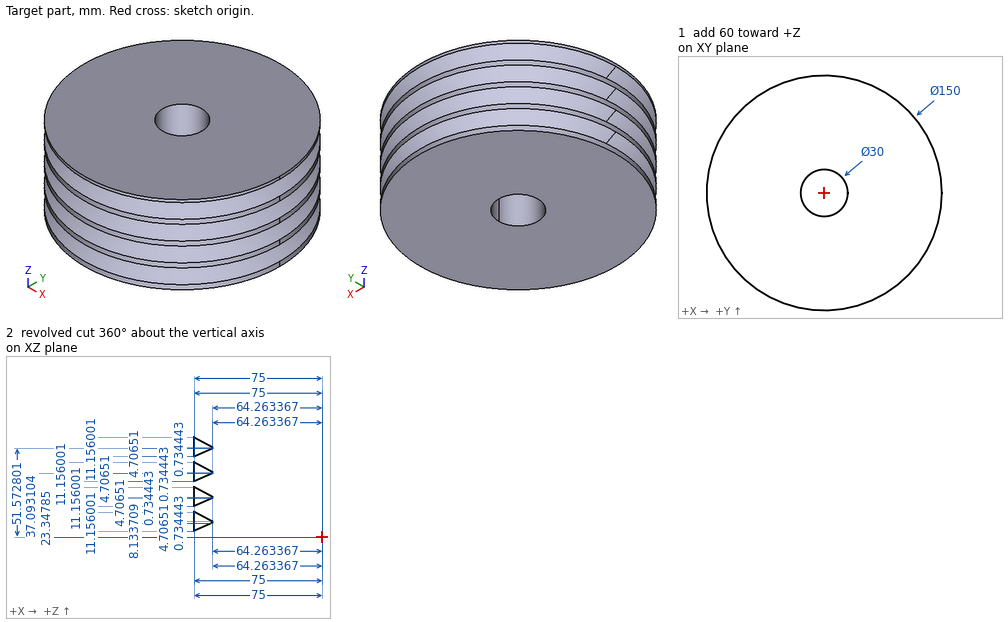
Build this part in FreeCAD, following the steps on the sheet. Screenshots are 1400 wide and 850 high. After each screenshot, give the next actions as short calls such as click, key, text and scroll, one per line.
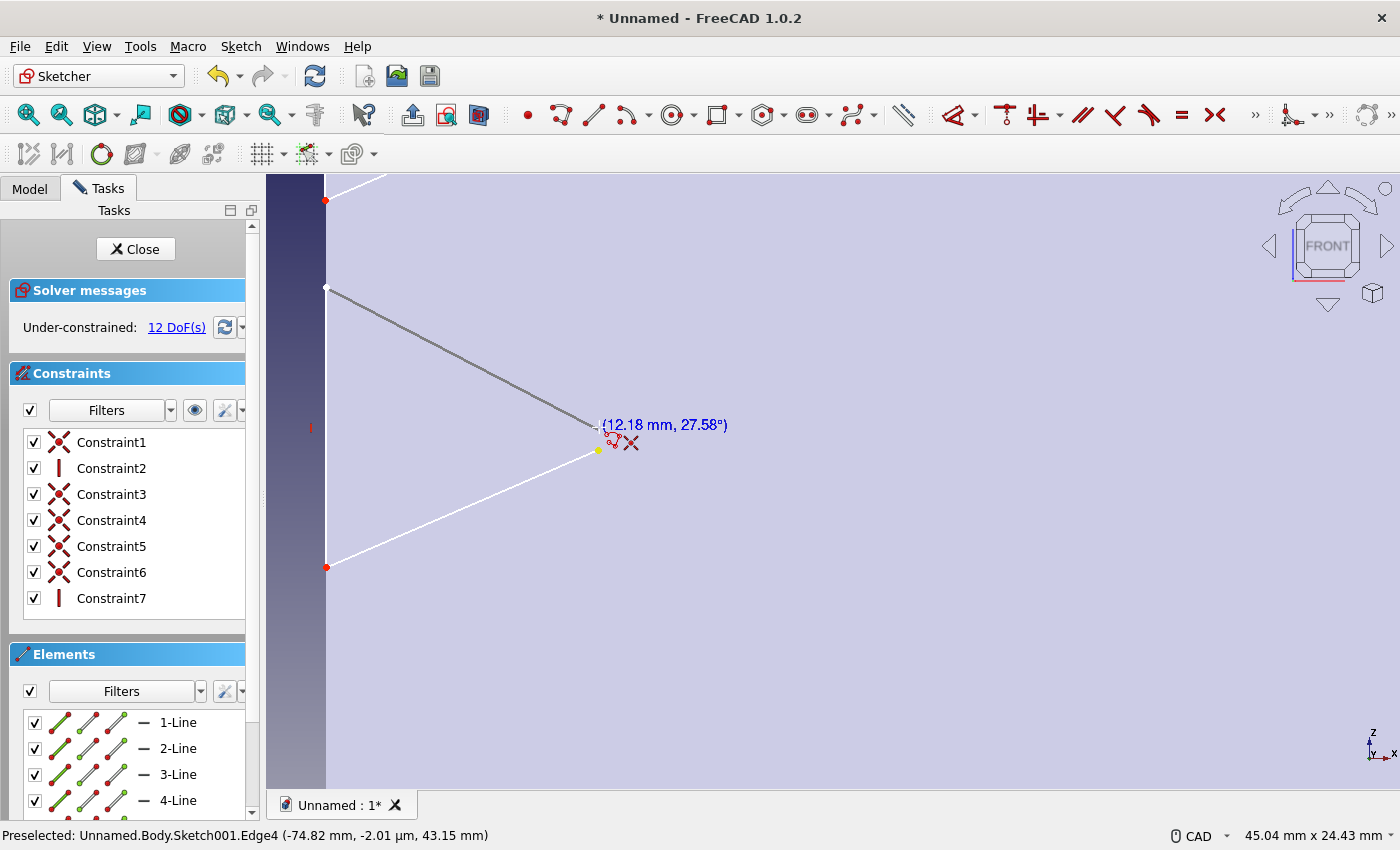
click(596, 426)
click(598, 450)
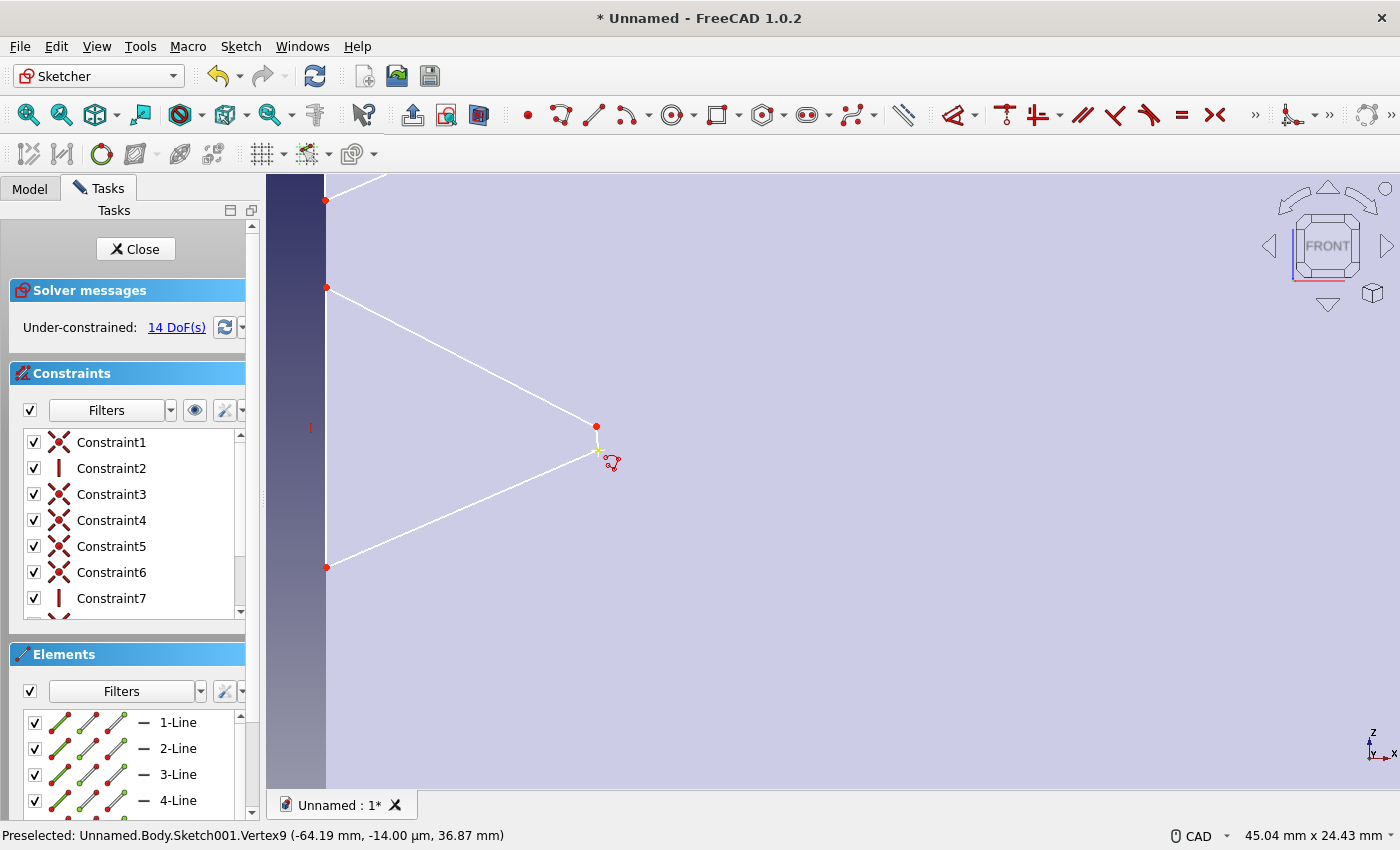
scroll(599, 427, down, 7)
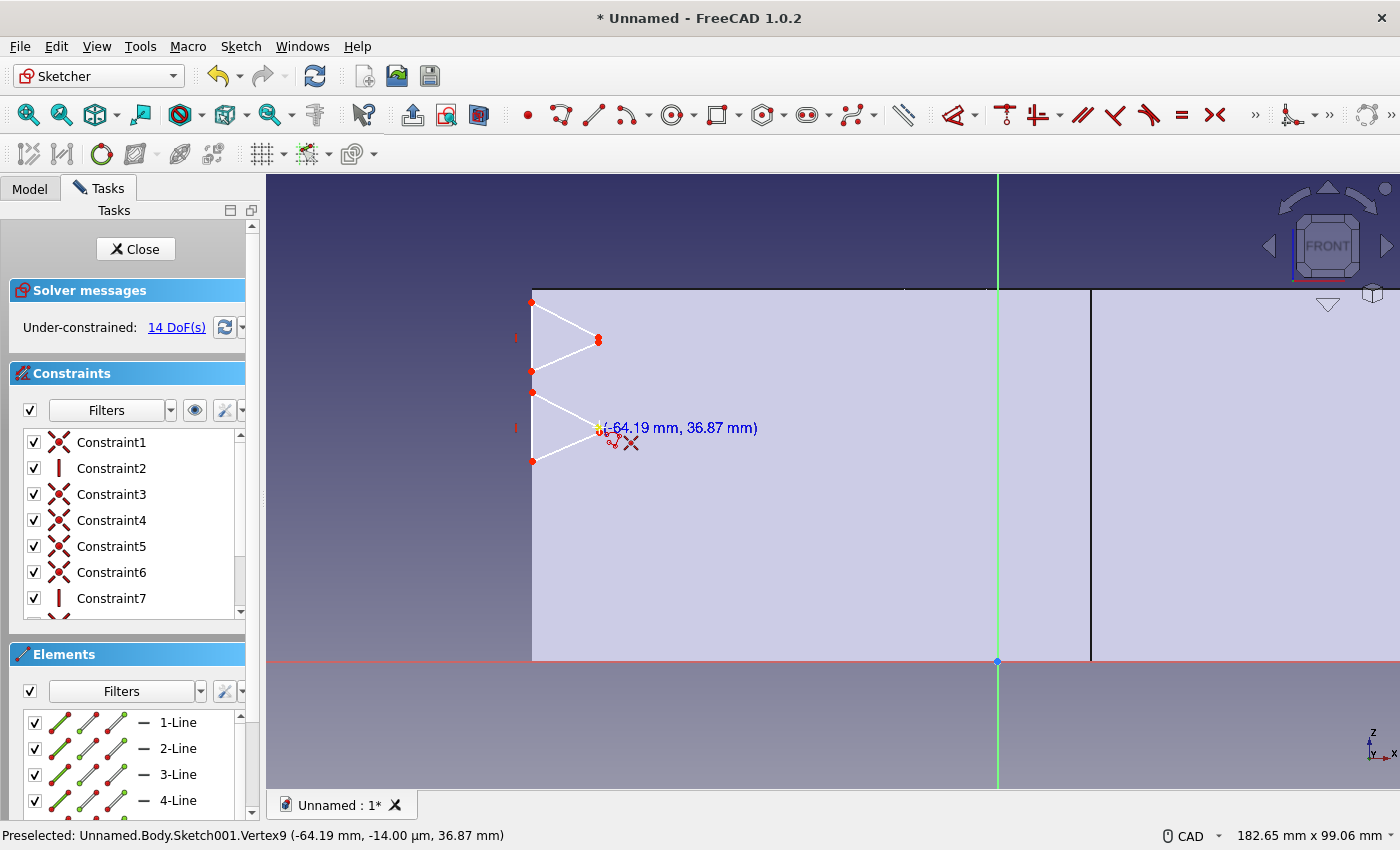
click(599, 522)
click(532, 551)
click(532, 481)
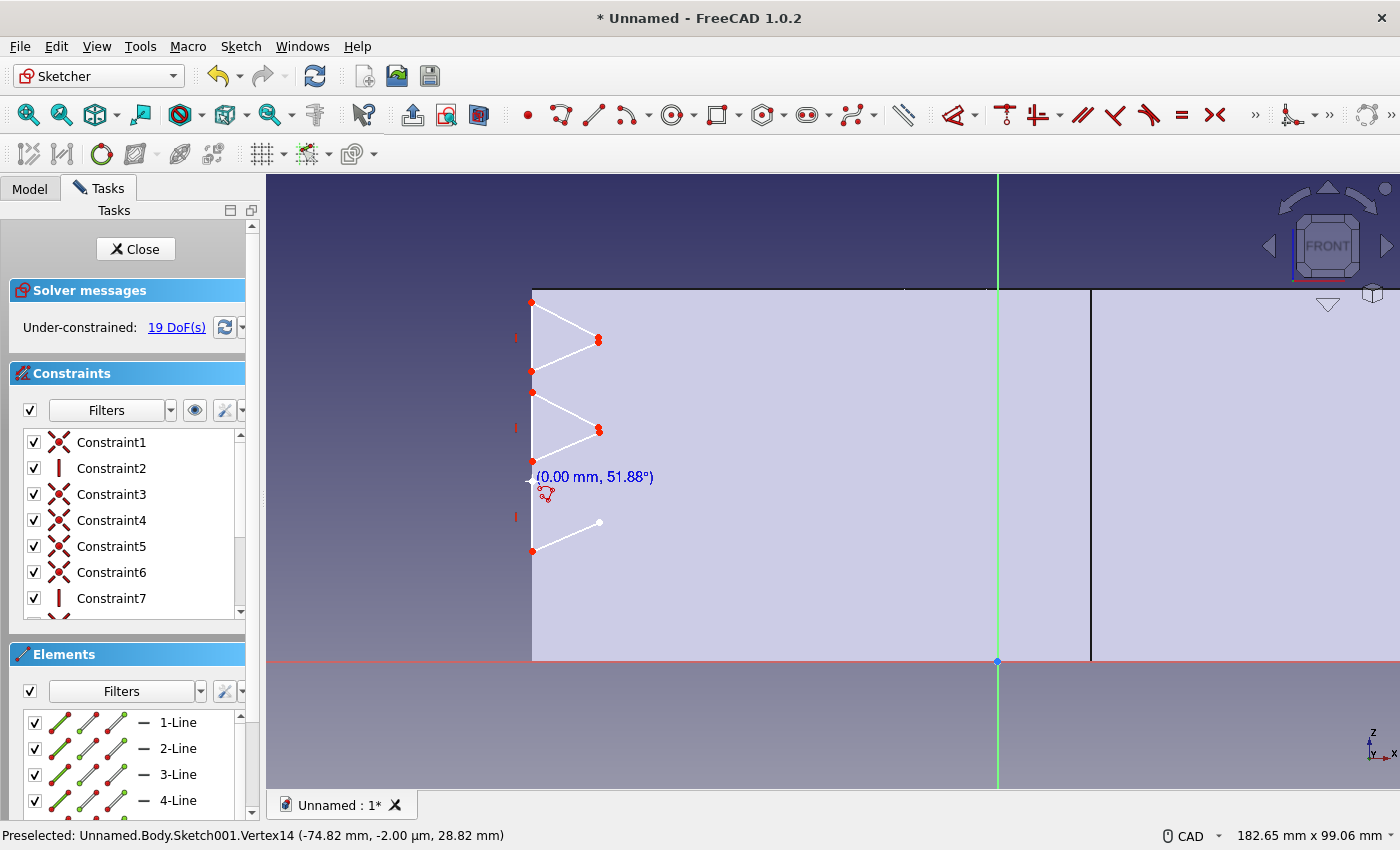
scroll(599, 517, up, 7)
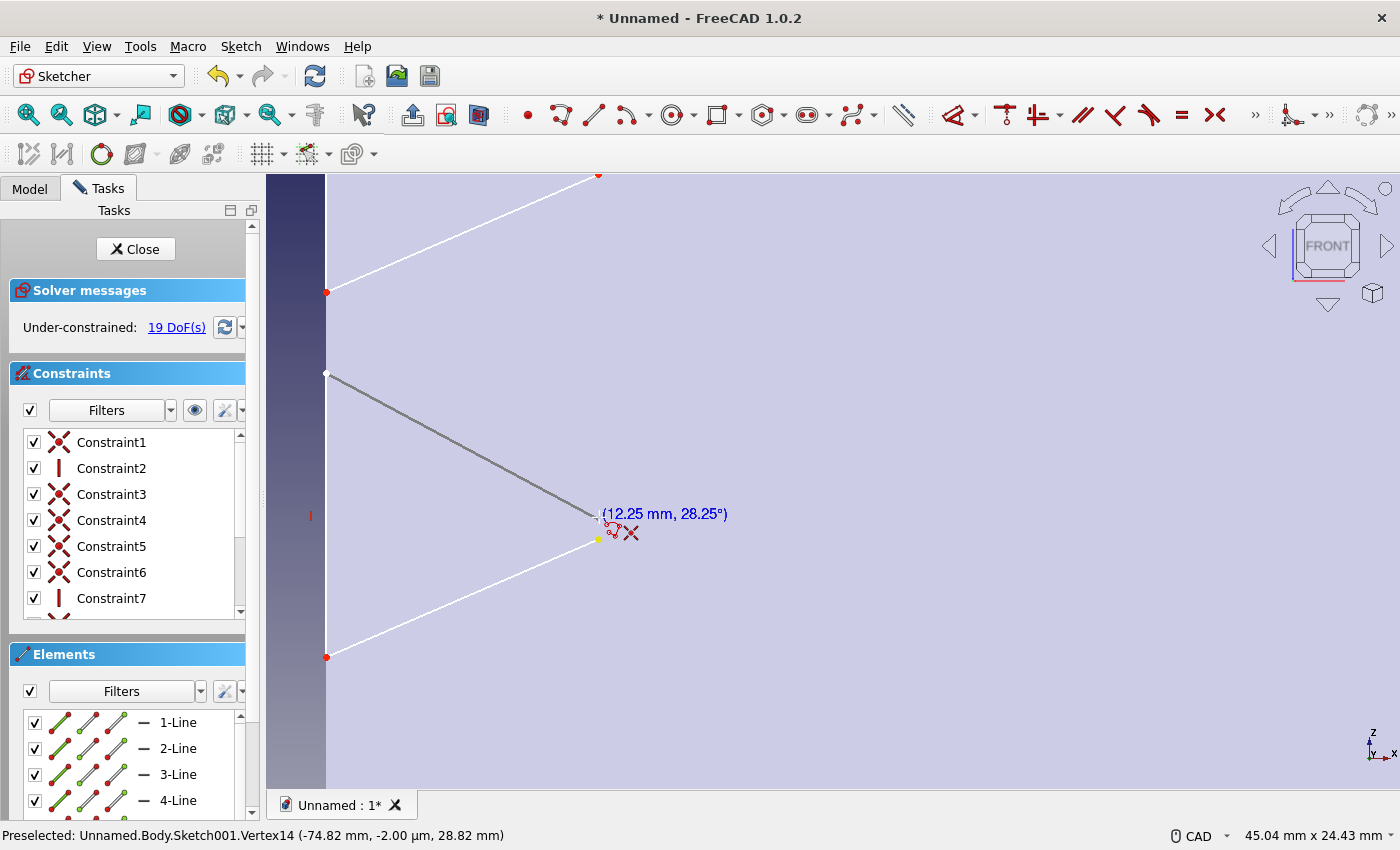
click(596, 515)
click(598, 540)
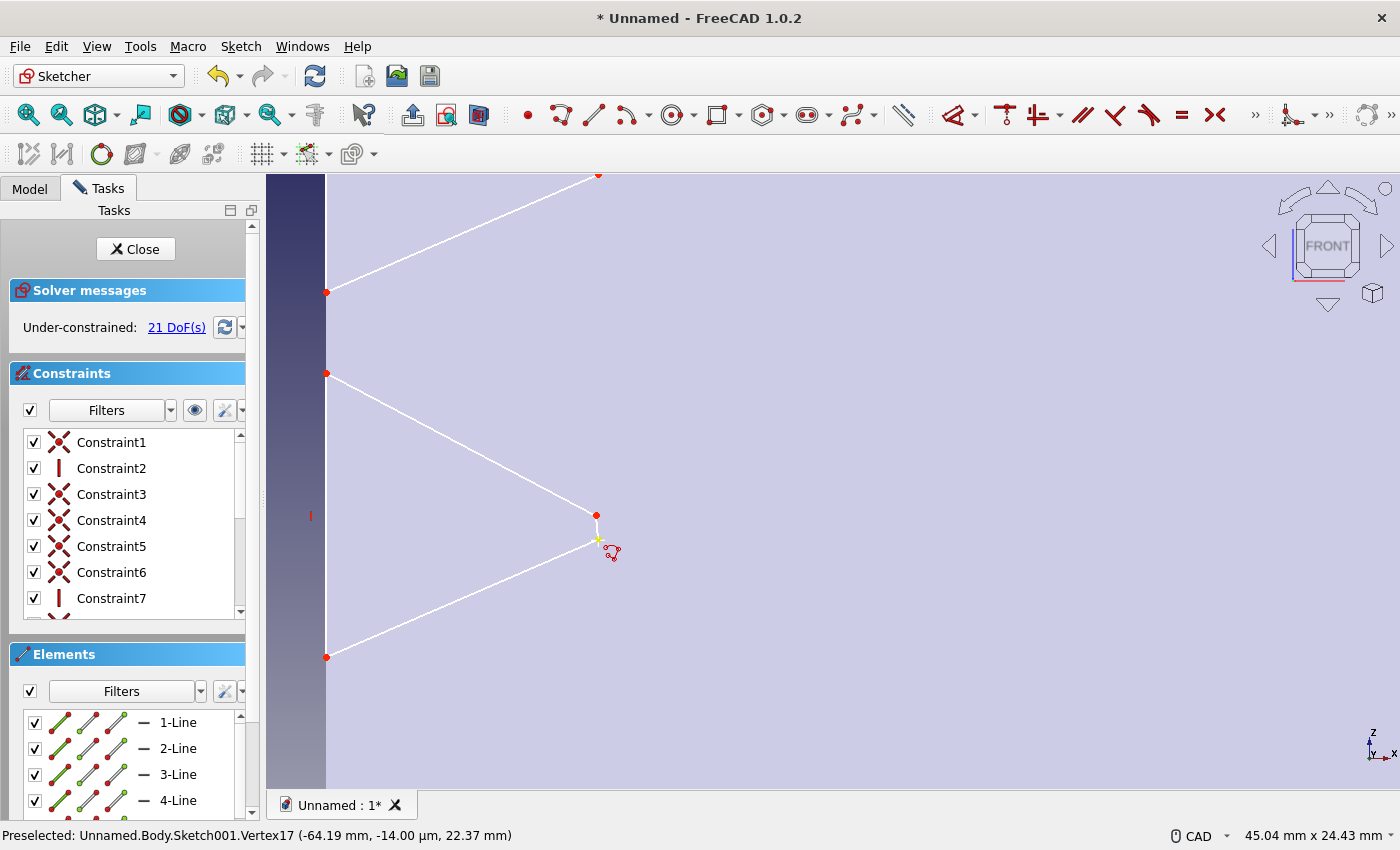
scroll(599, 517, down, 7)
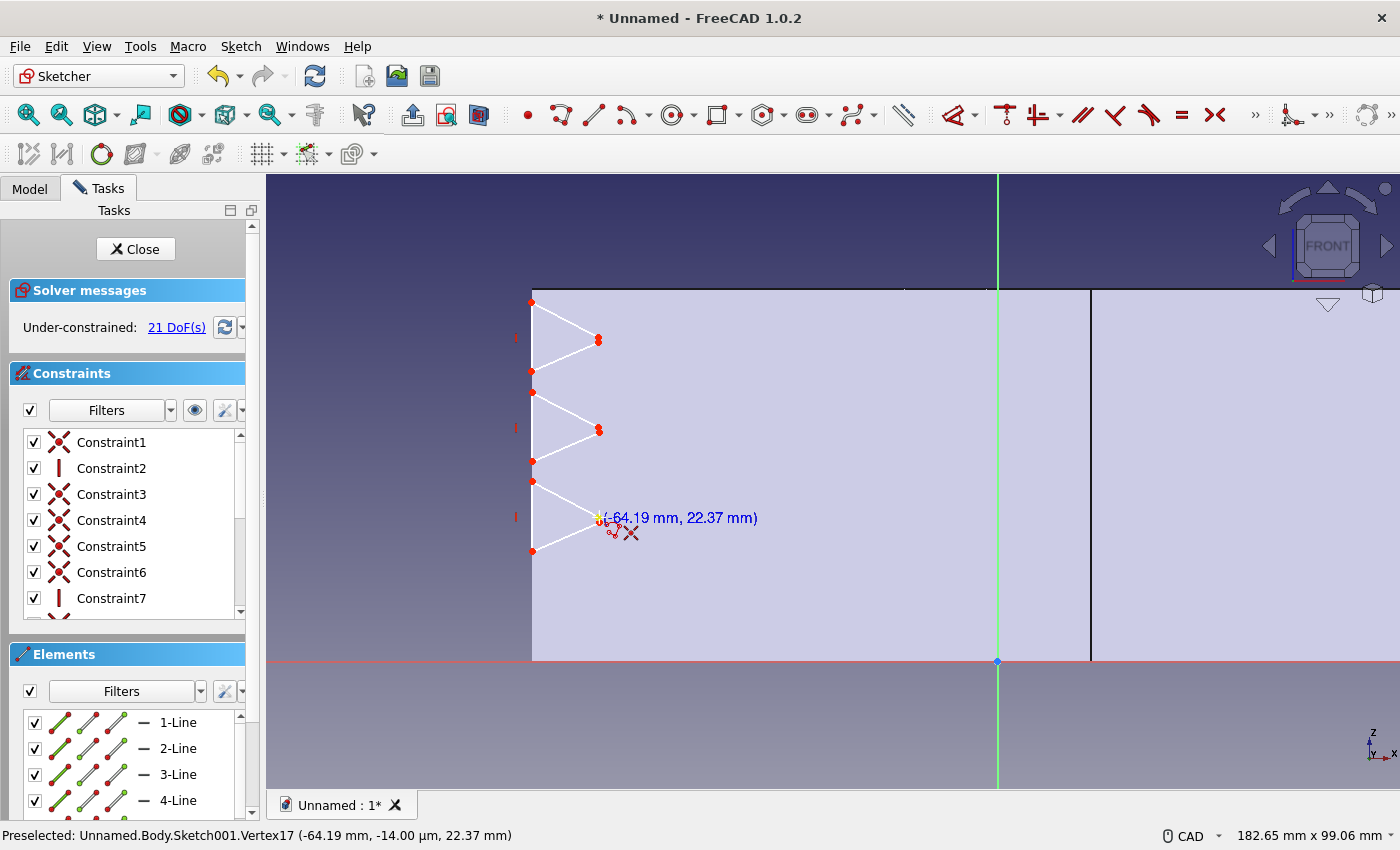
click(599, 611)
click(532, 641)
click(532, 571)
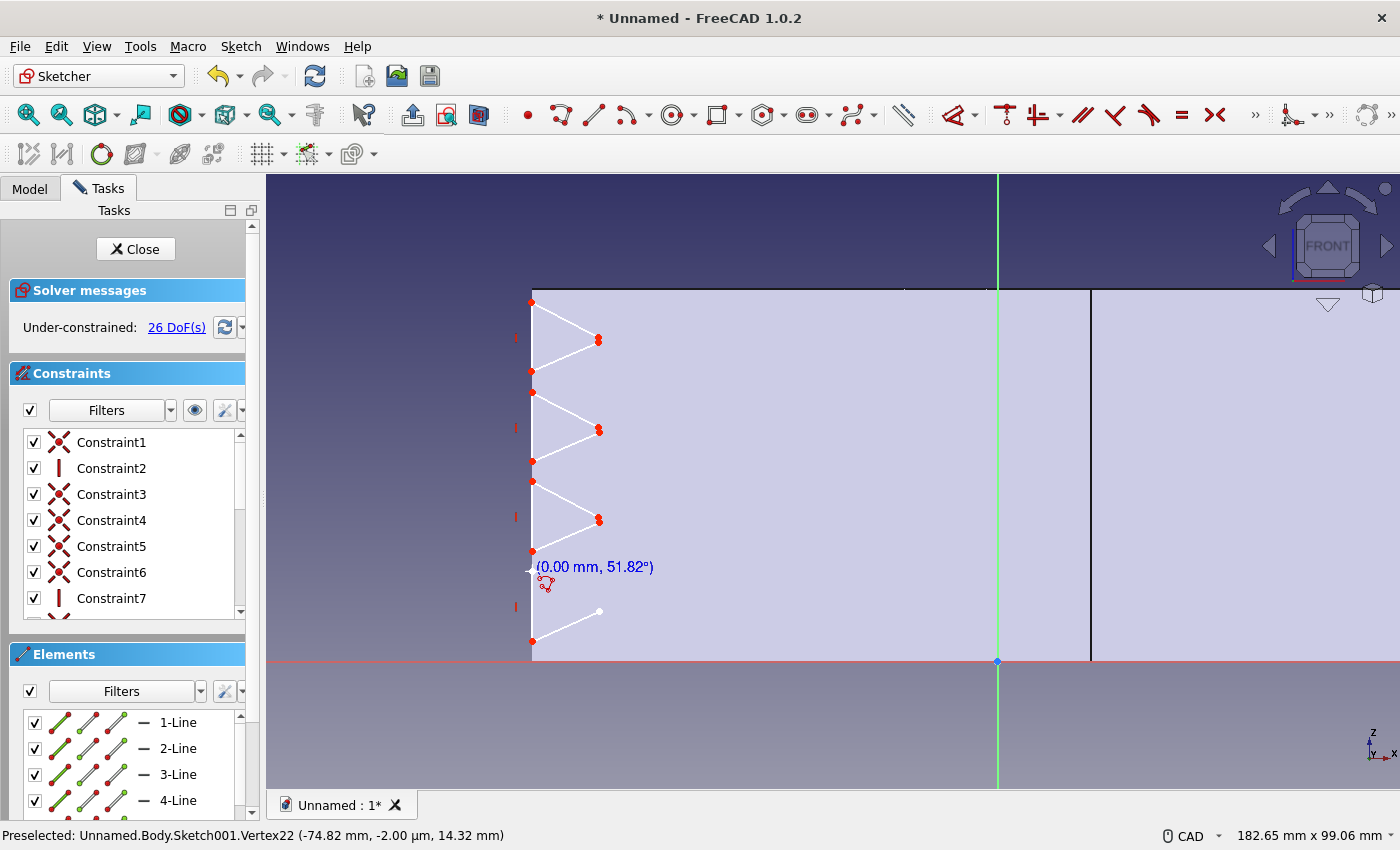
scroll(599, 607, up, 7)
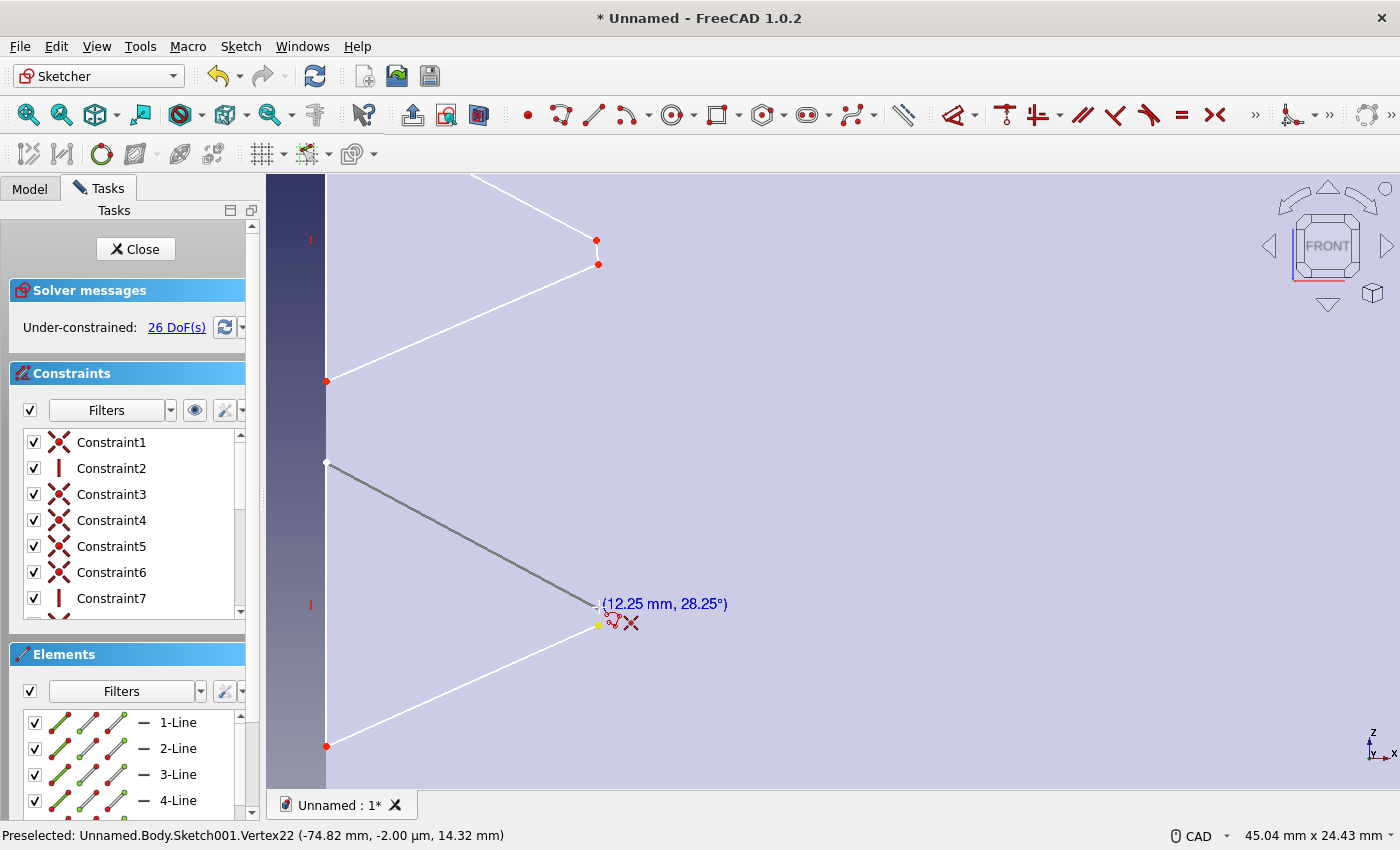
click(596, 604)
click(598, 625)
key(Escape)
key(Escape)